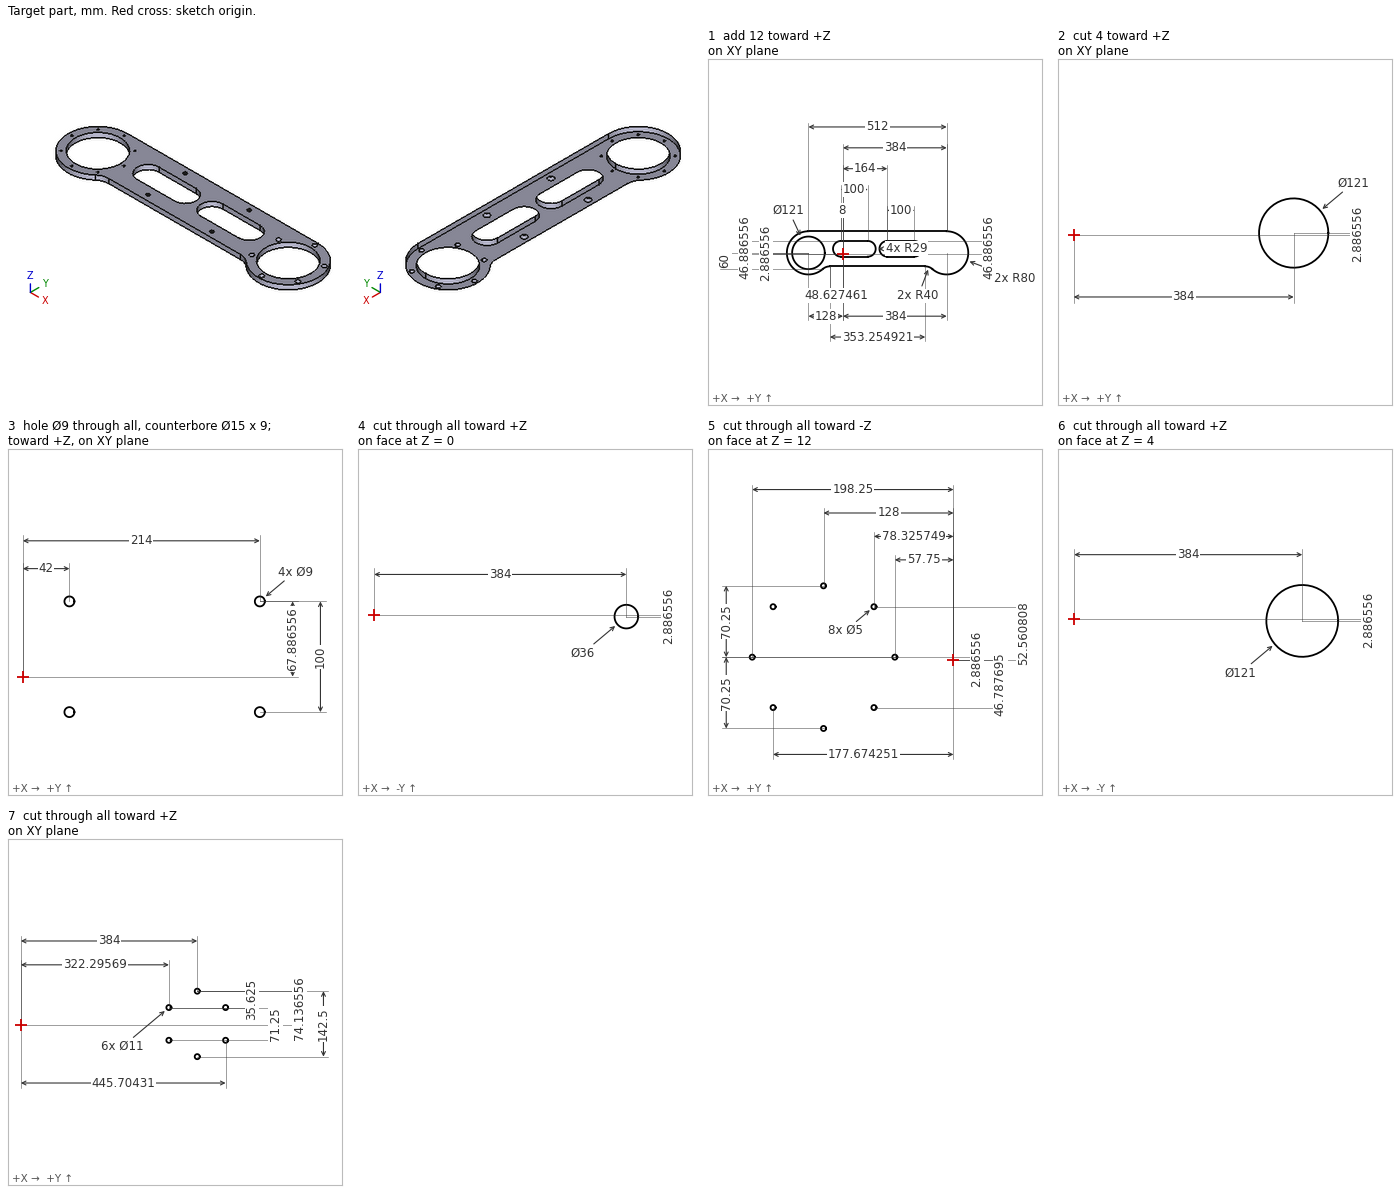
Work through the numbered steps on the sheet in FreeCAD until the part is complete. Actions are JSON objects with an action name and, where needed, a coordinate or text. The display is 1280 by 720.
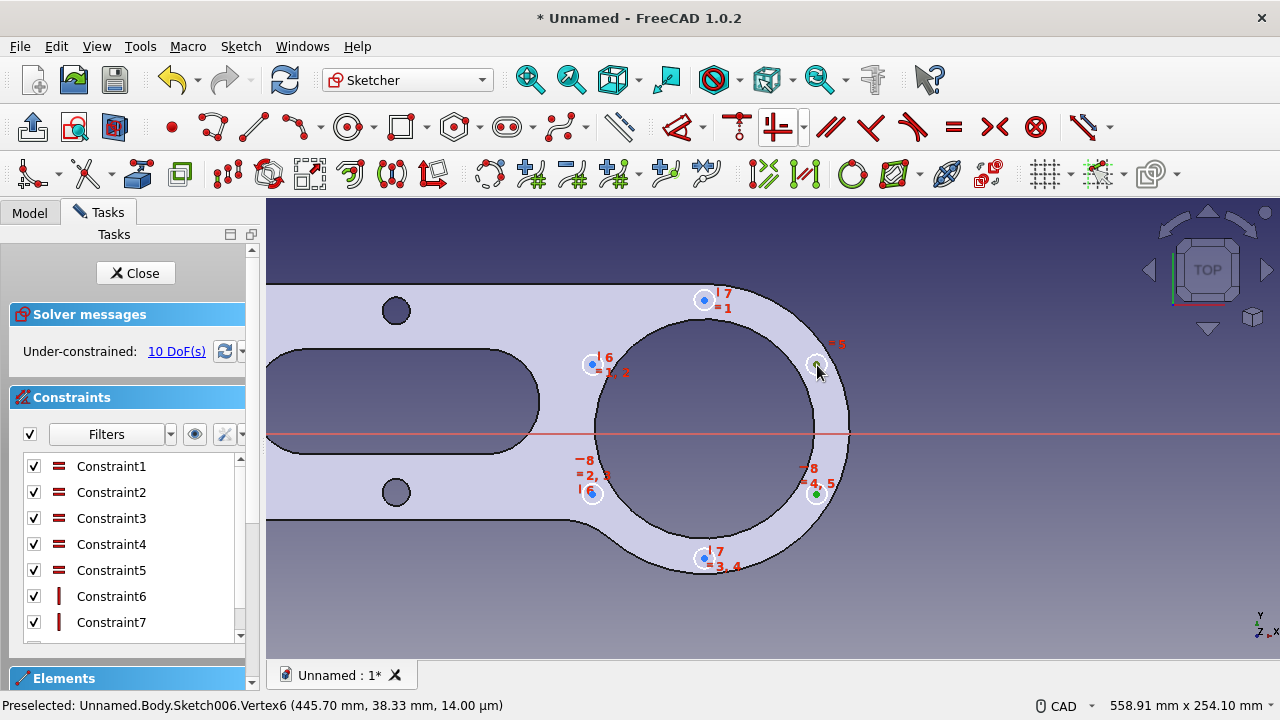
{"action": "left_click", "coordinate": [804, 128]}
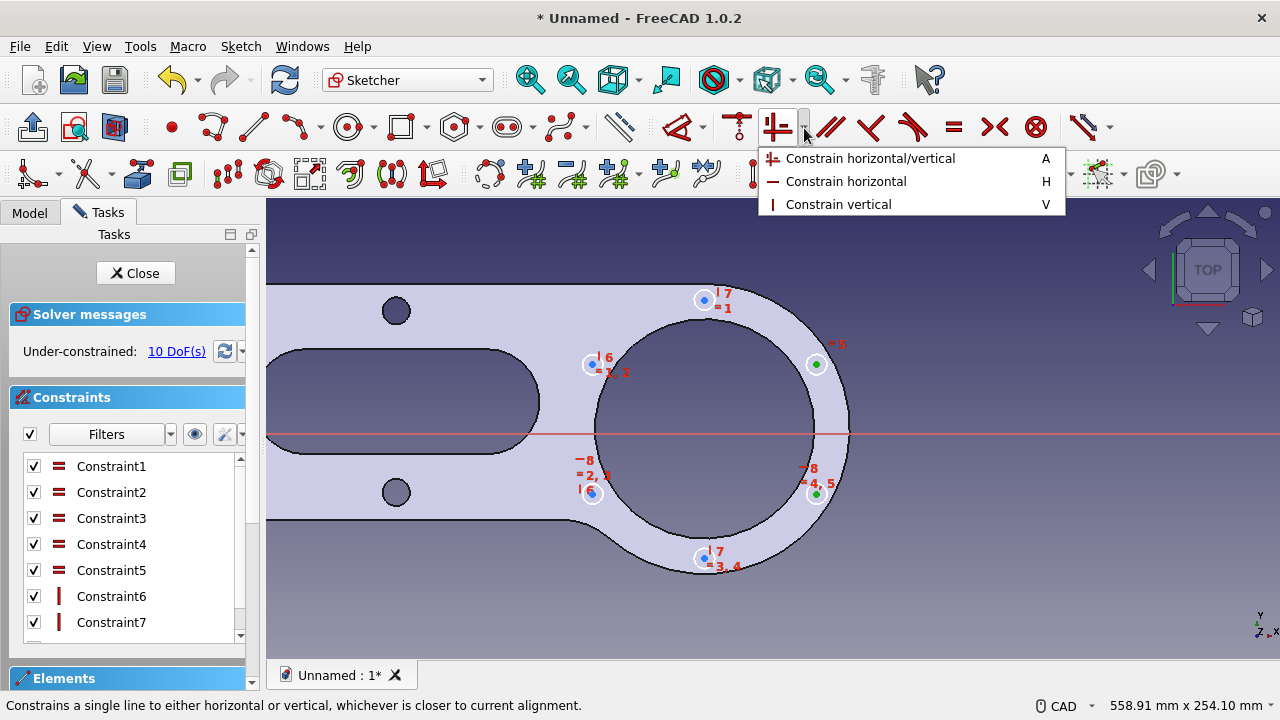
{"action": "left_click", "coordinate": [912, 204]}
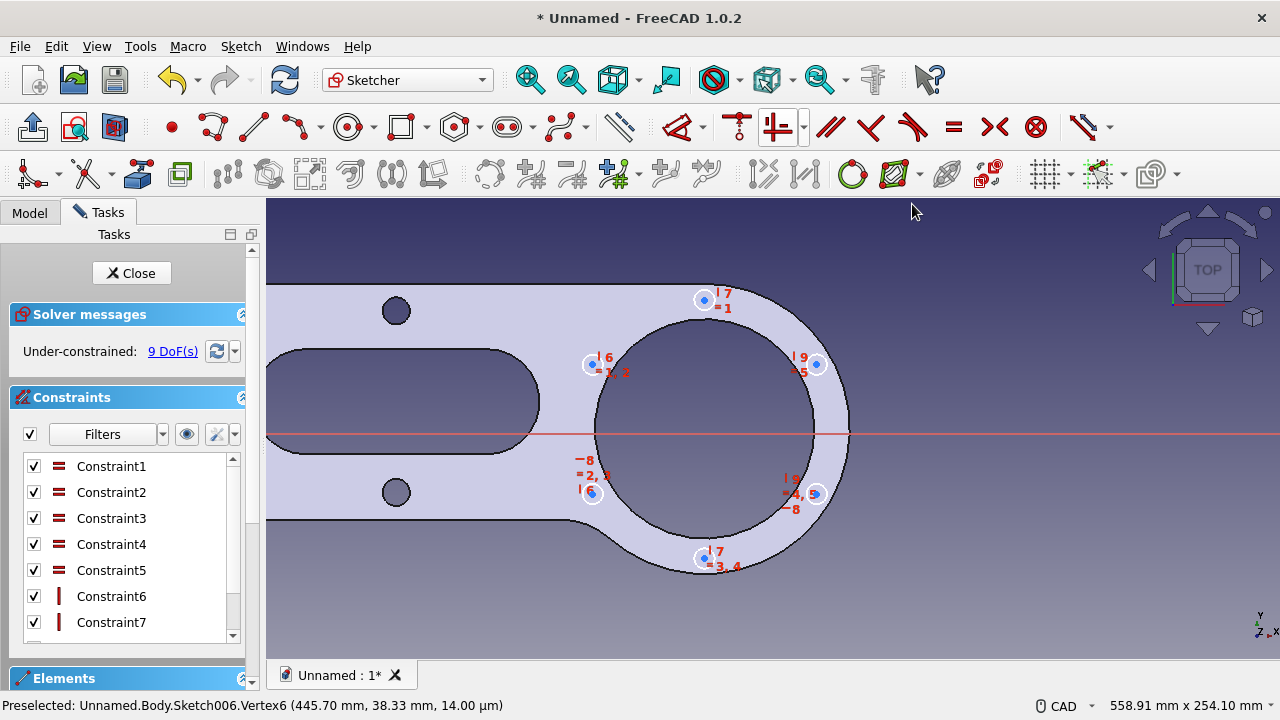
{"action": "left_click", "coordinate": [593, 365]}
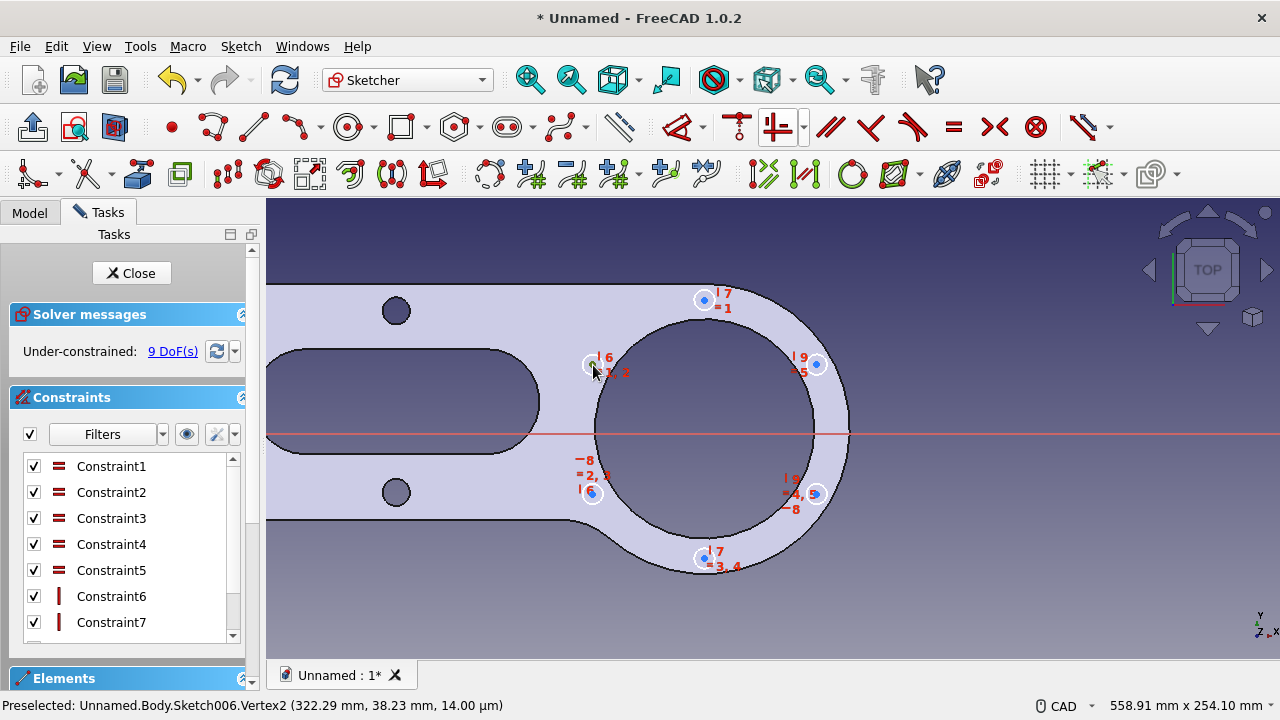
{"action": "left_click", "coordinate": [817, 365]}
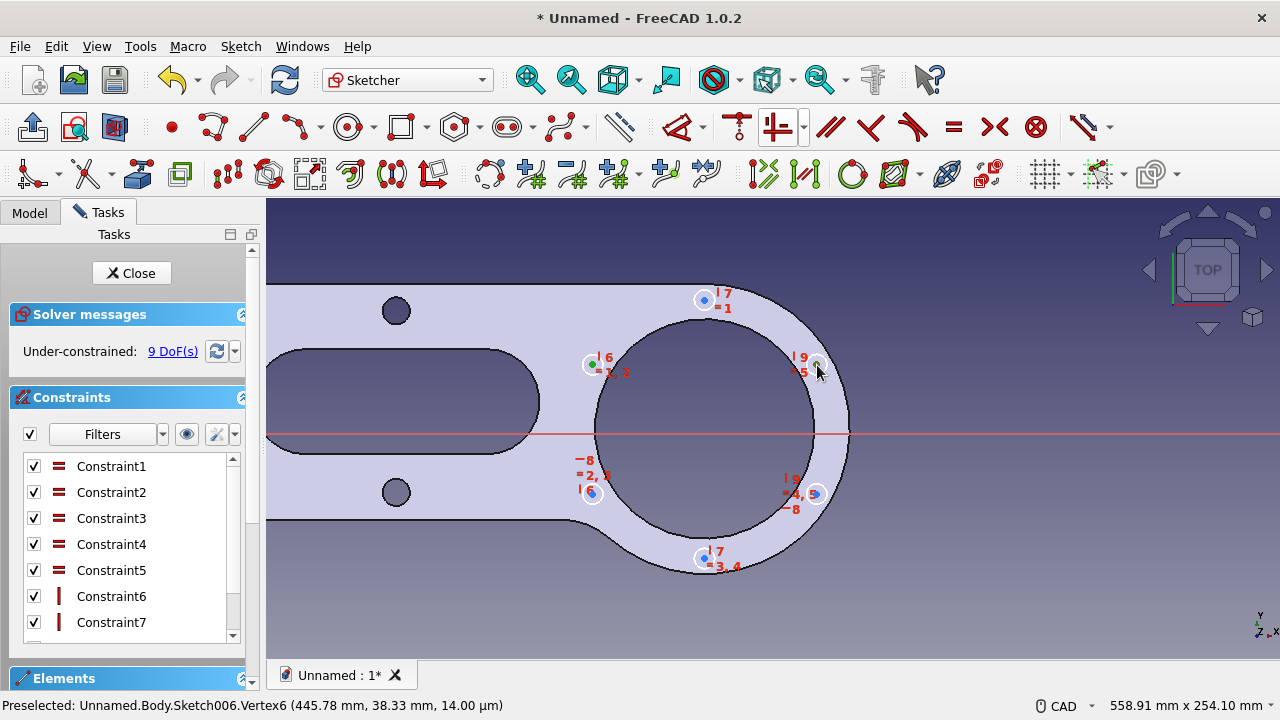
{"action": "key", "text": "h"}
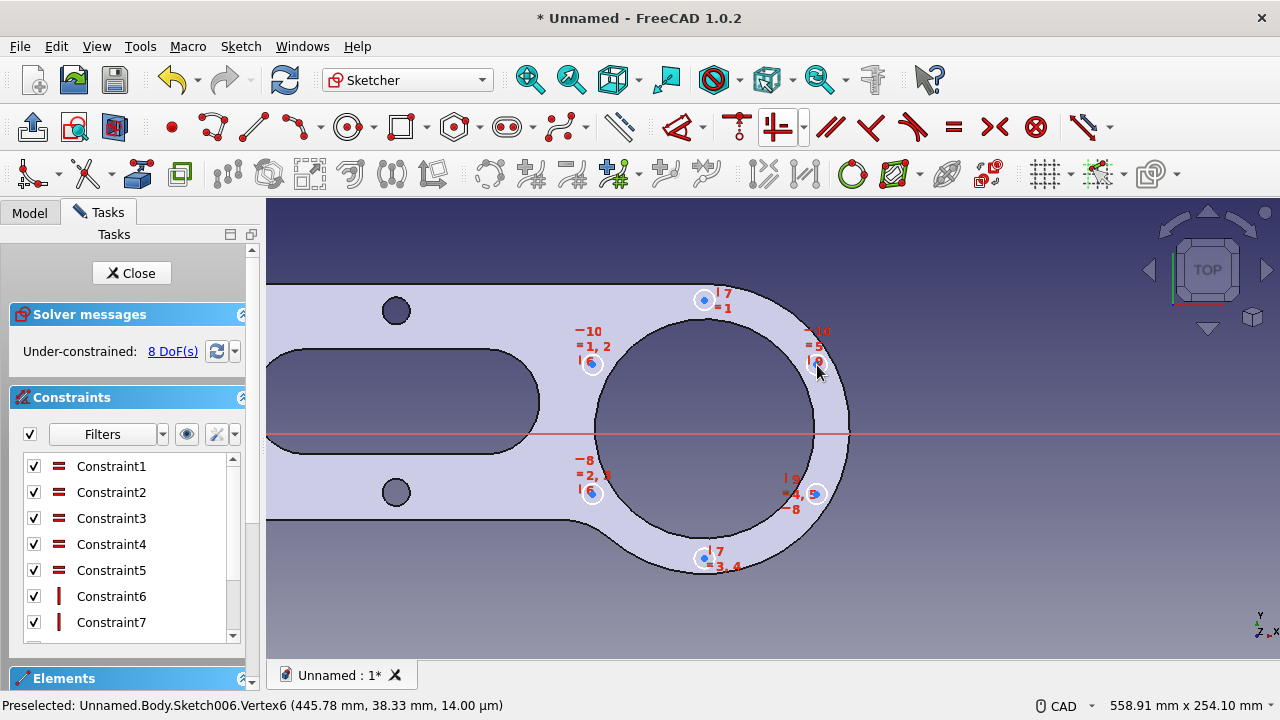
{"action": "left_click", "coordinate": [676, 128]}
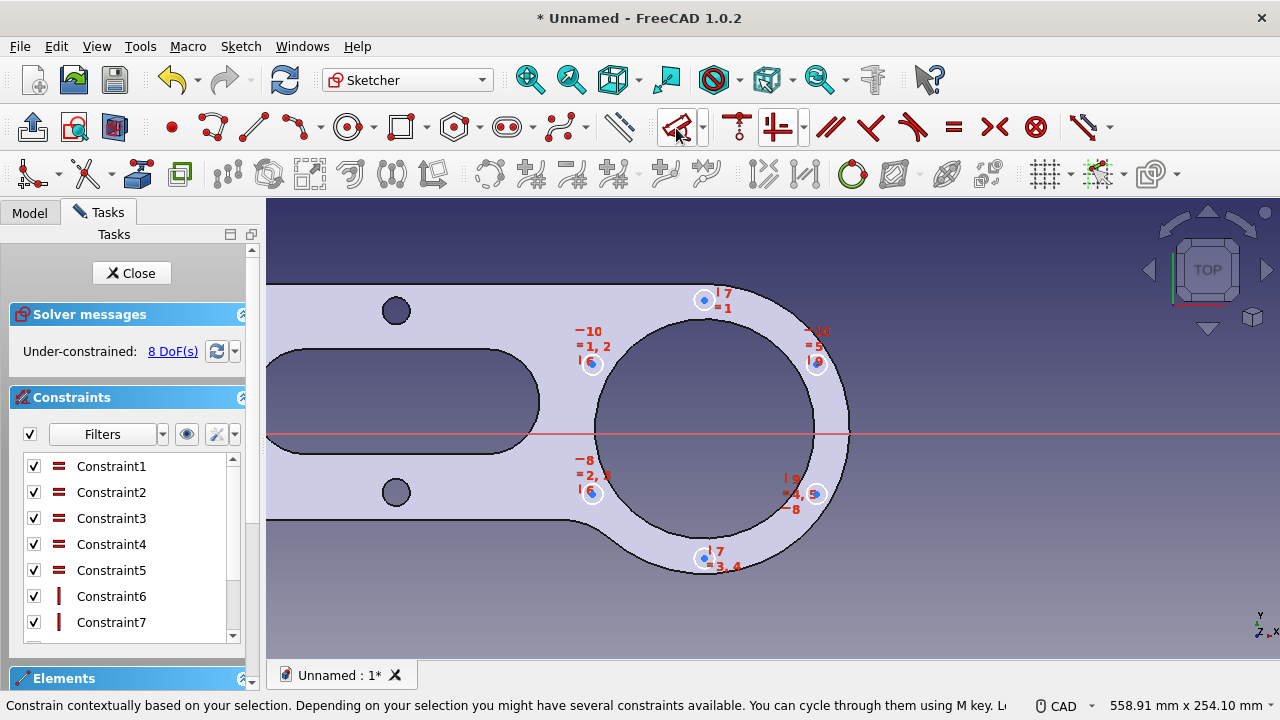
{"action": "scroll", "coordinate": [712, 293], "scroll_direction": "up", "scroll_amount": 4}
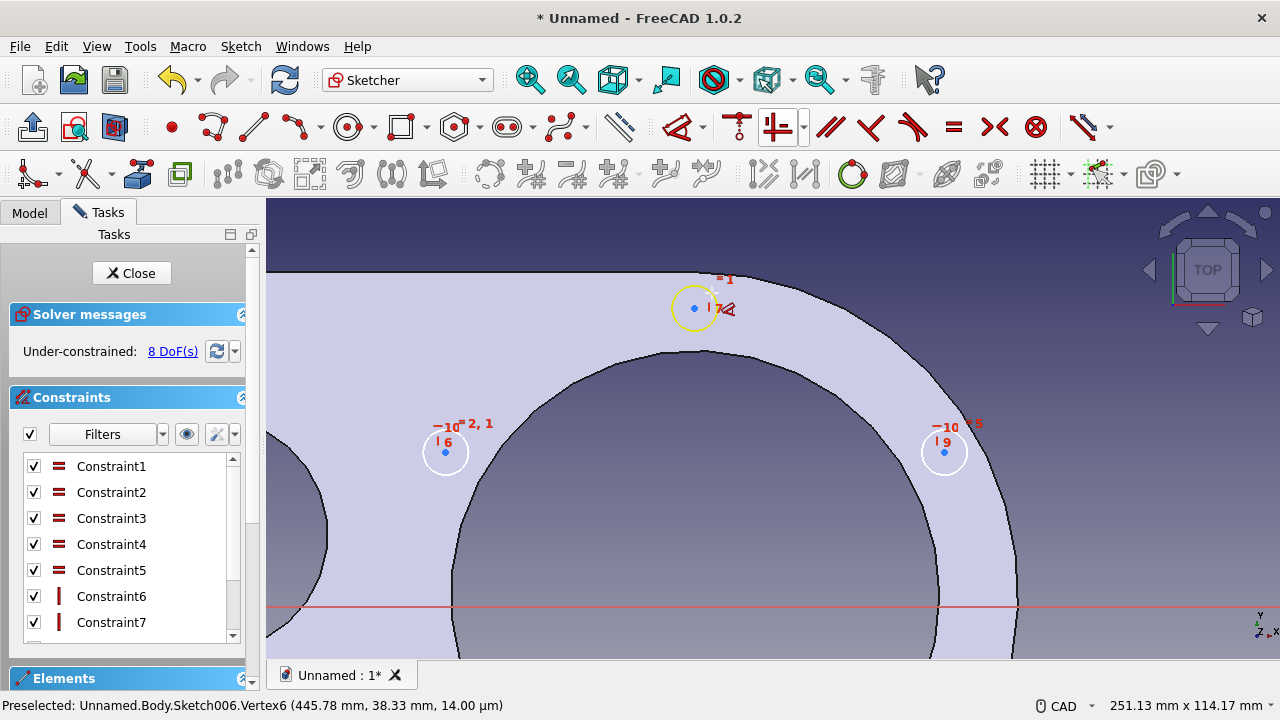
{"action": "left_click", "coordinate": [711, 292]}
{"action": "left_click", "coordinate": [733, 269]}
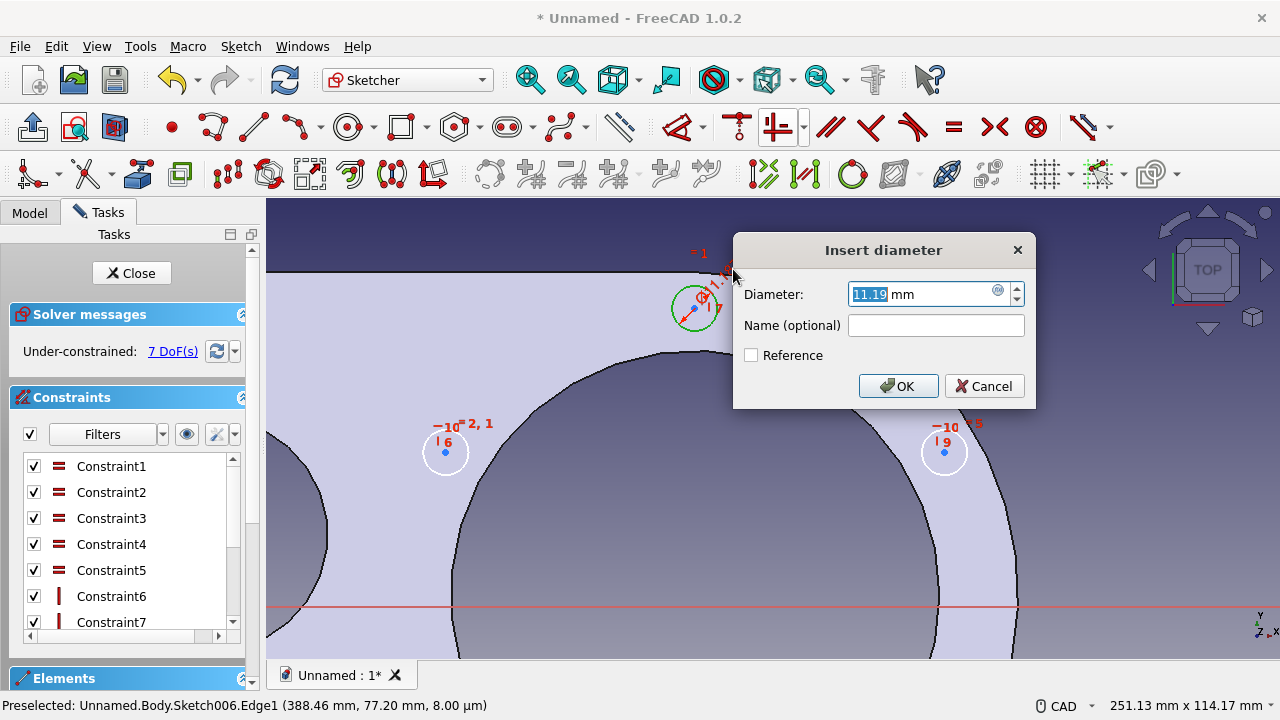
{"action": "type", "text": "11"}
{"action": "key", "text": "Return"}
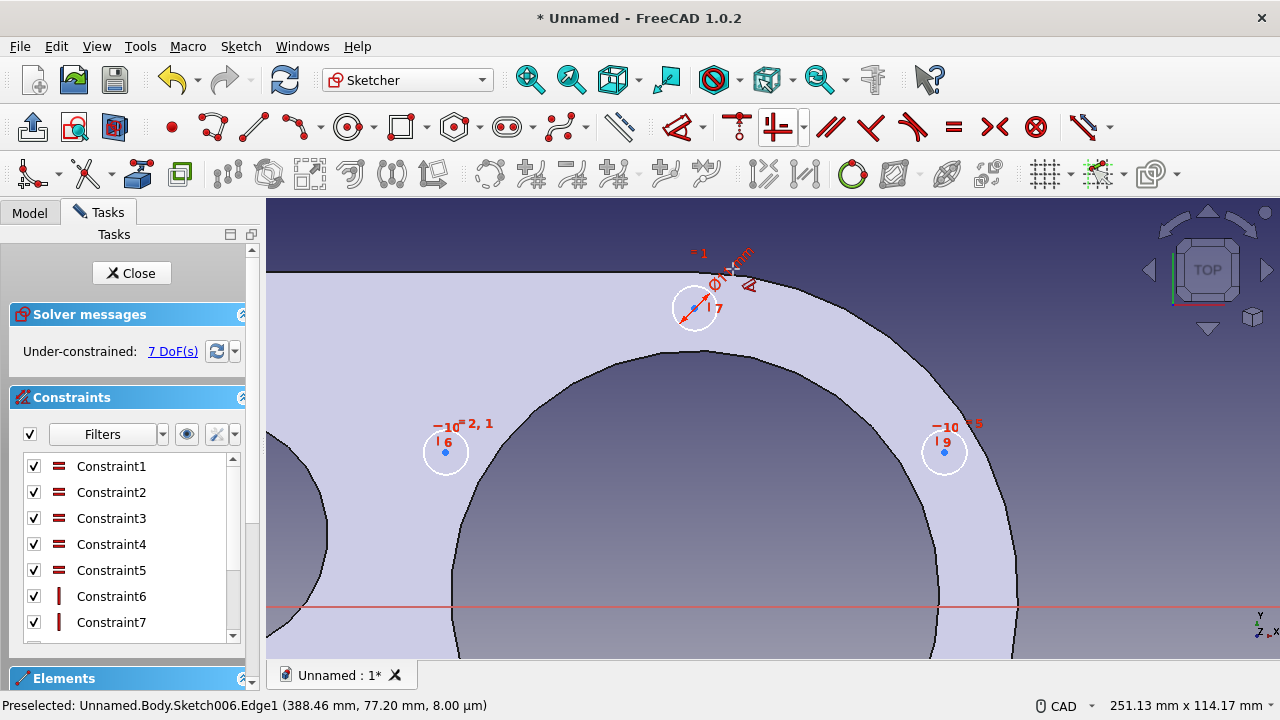
{"action": "left_click", "coordinate": [695, 308]}
{"action": "left_click", "coordinate": [494, 274]}